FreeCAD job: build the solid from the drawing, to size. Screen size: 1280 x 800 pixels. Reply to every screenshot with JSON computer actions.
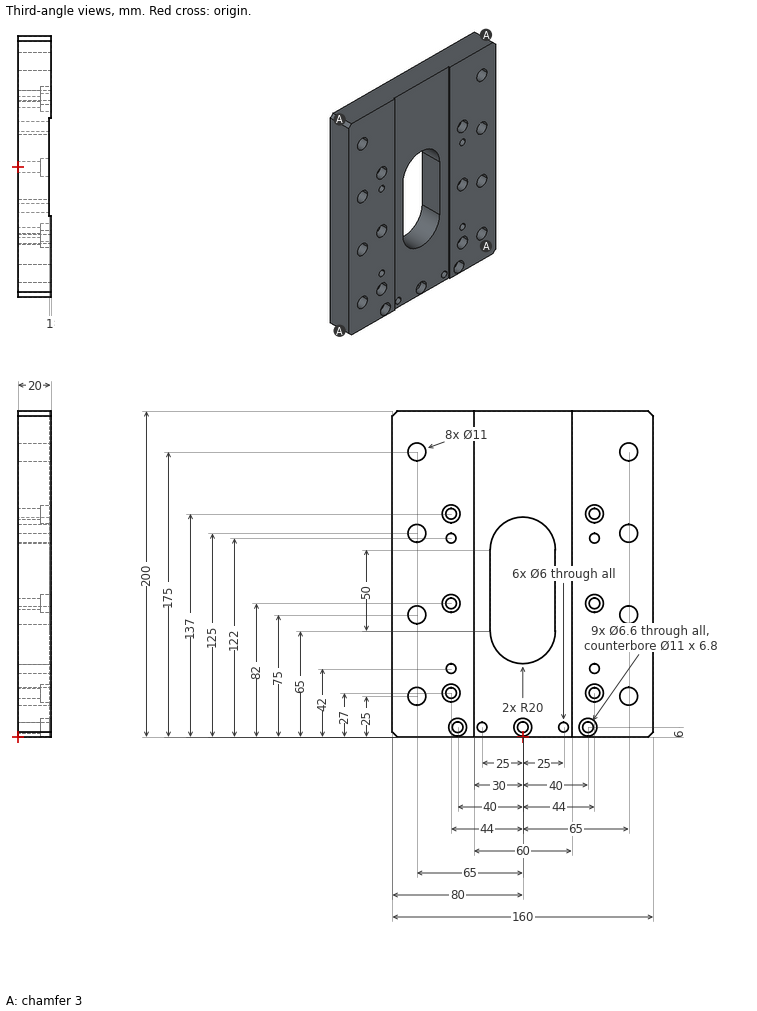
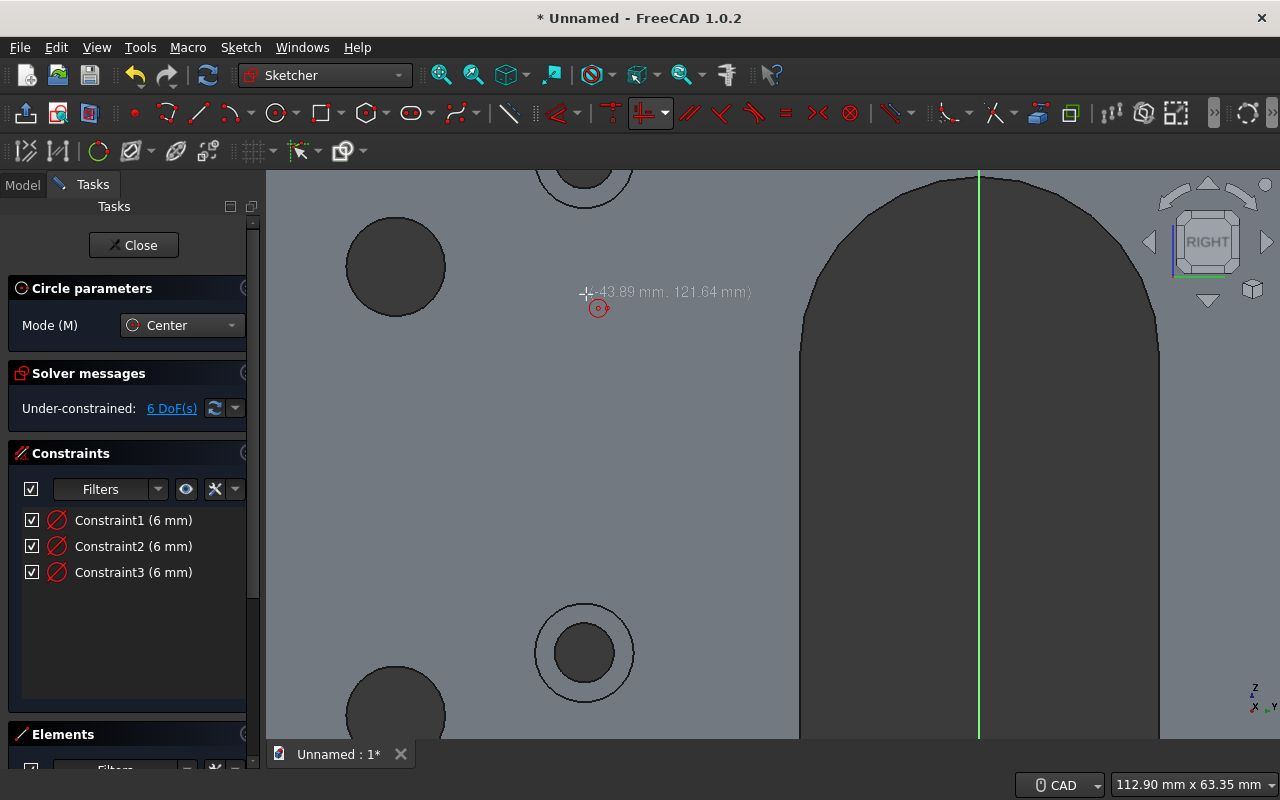
{"action": "scroll", "coordinate": [586, 294], "scroll_direction": "down", "scroll_amount": 6}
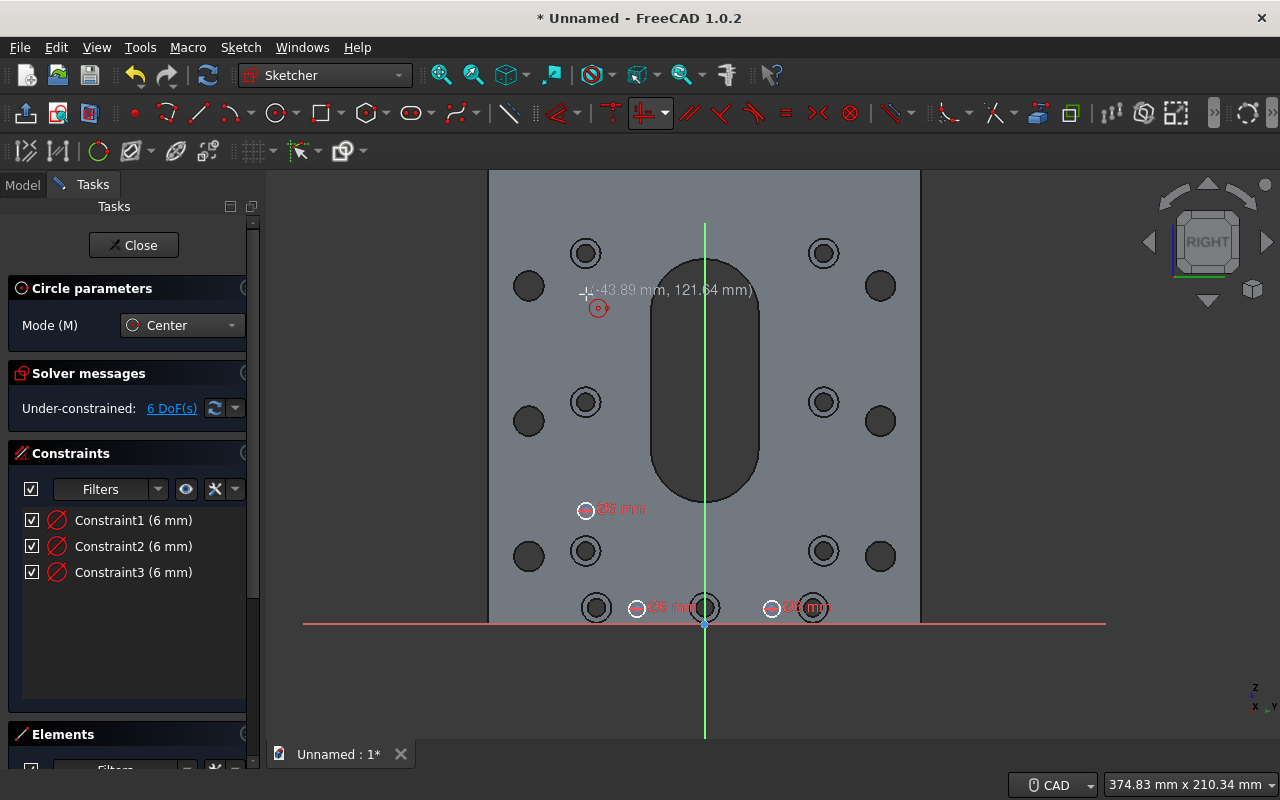
{"action": "left_click", "coordinate": [586, 294]}
{"action": "mouse_move", "coordinate": [591, 288]}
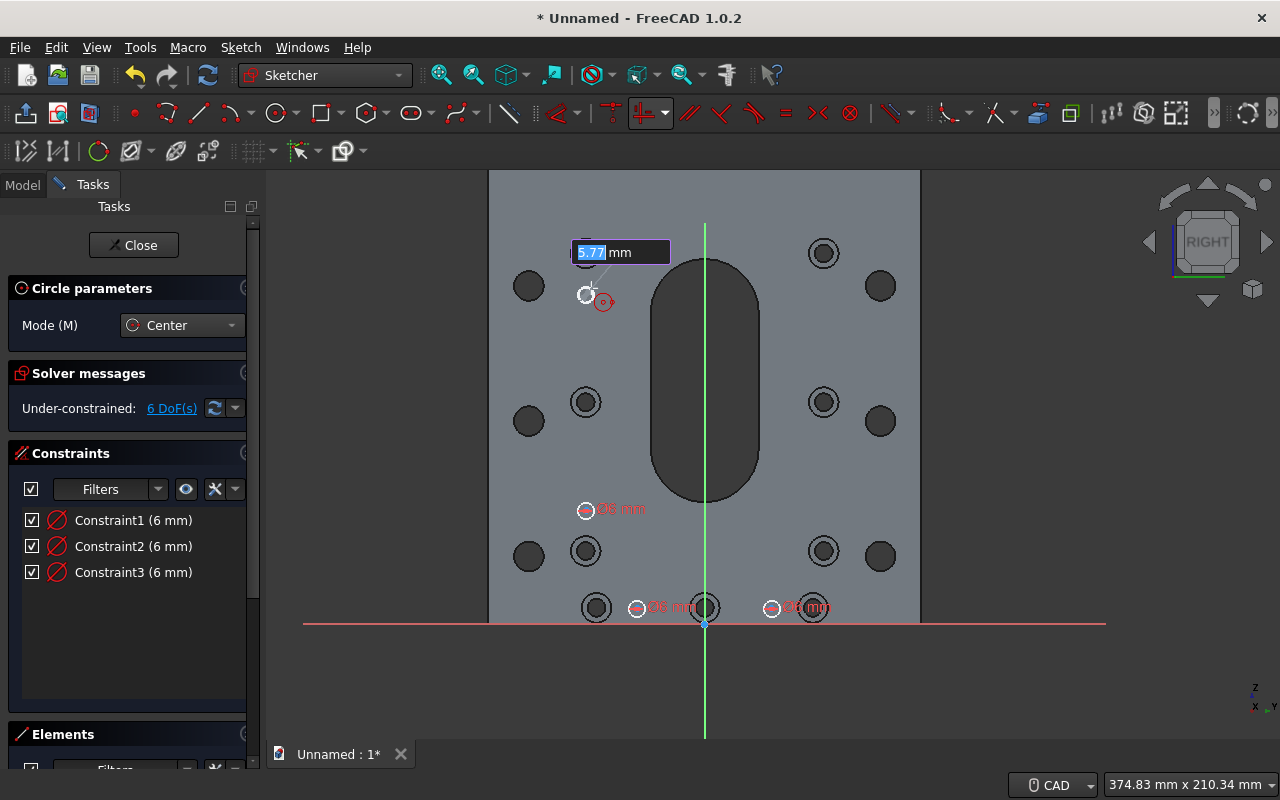
{"action": "type", "text": "6"}
{"action": "key", "text": "Return"}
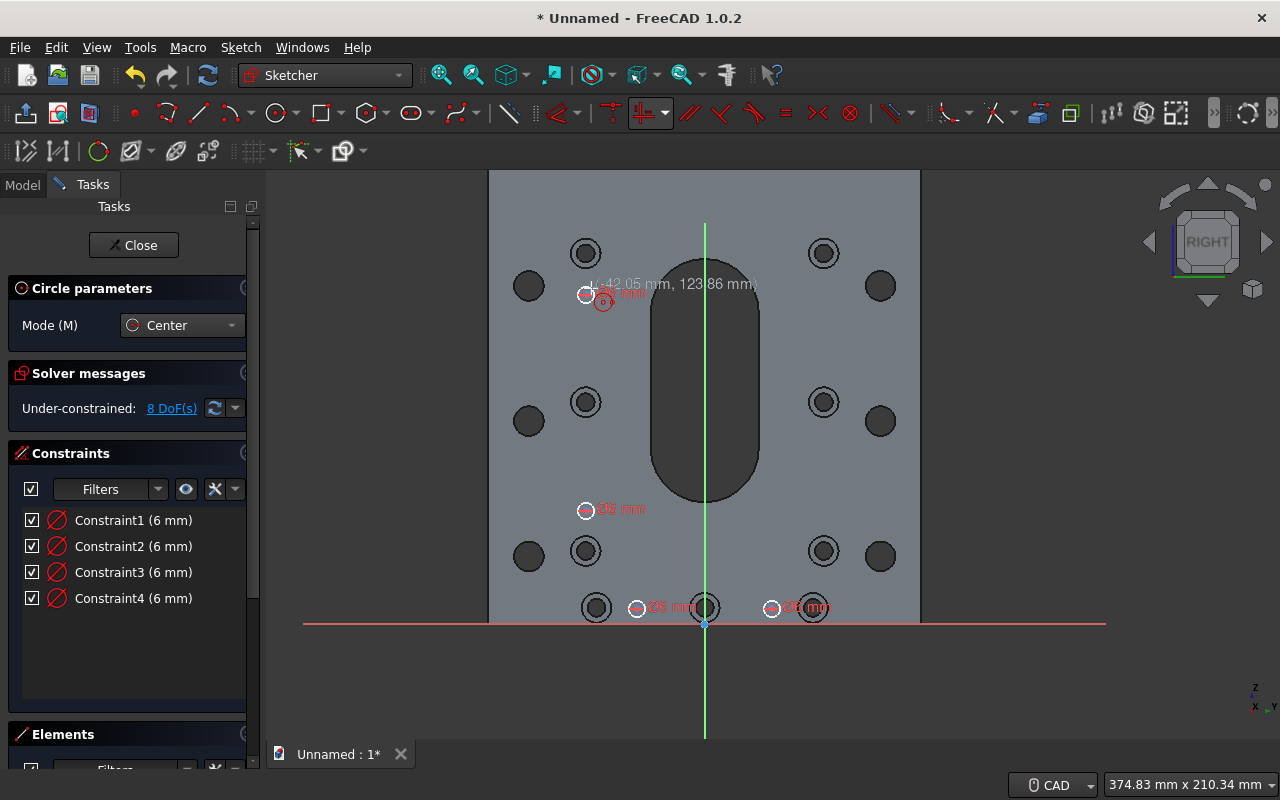
{"action": "scroll", "coordinate": [824, 294], "scroll_direction": "up", "scroll_amount": 6}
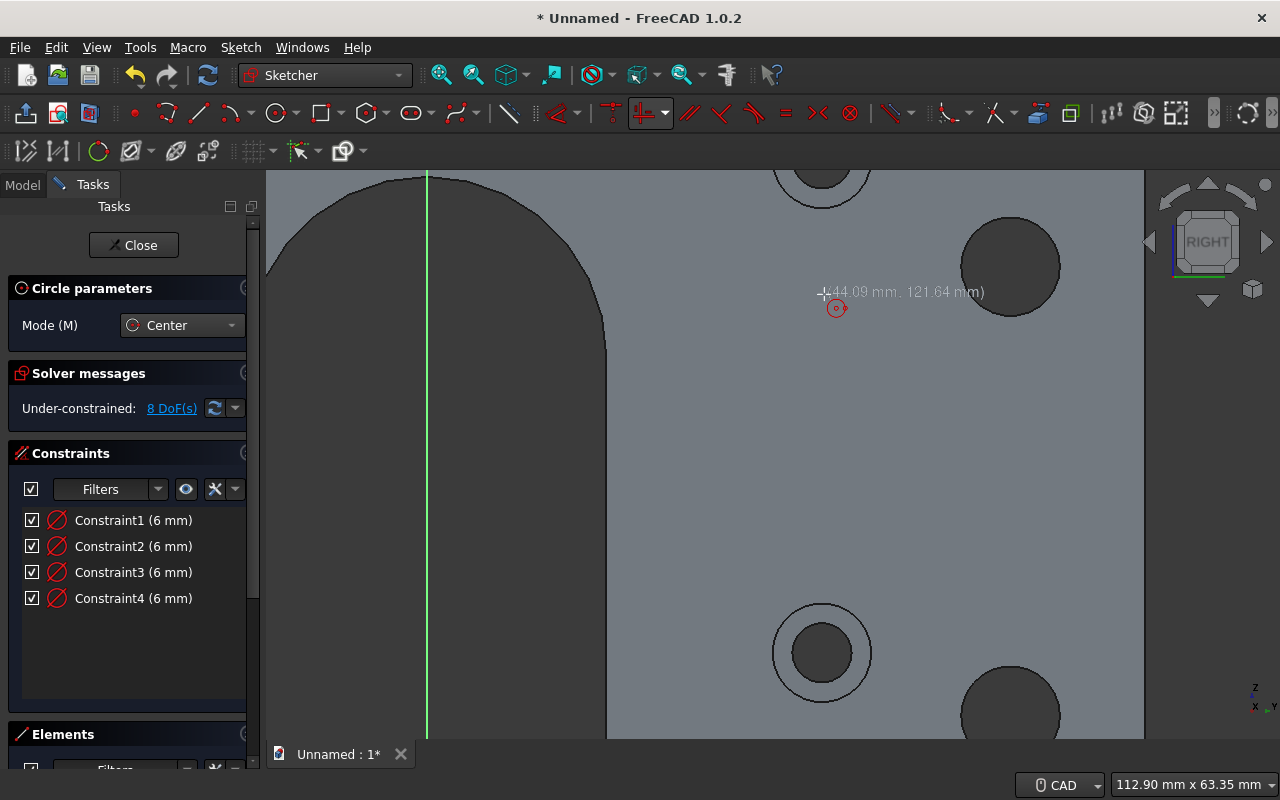
{"action": "scroll", "coordinate": [824, 294], "scroll_direction": "down", "scroll_amount": 6}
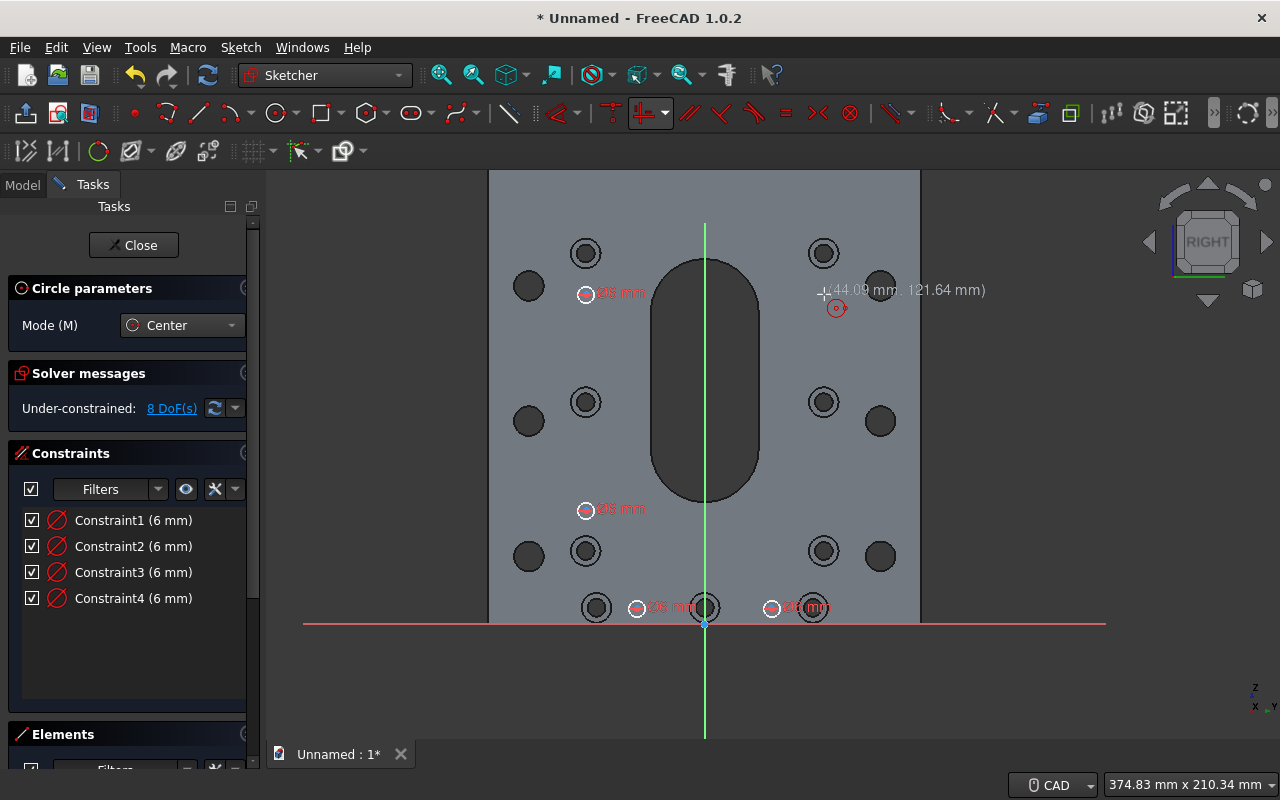
{"action": "left_click", "coordinate": [824, 294]}
{"action": "mouse_move", "coordinate": [830, 288]}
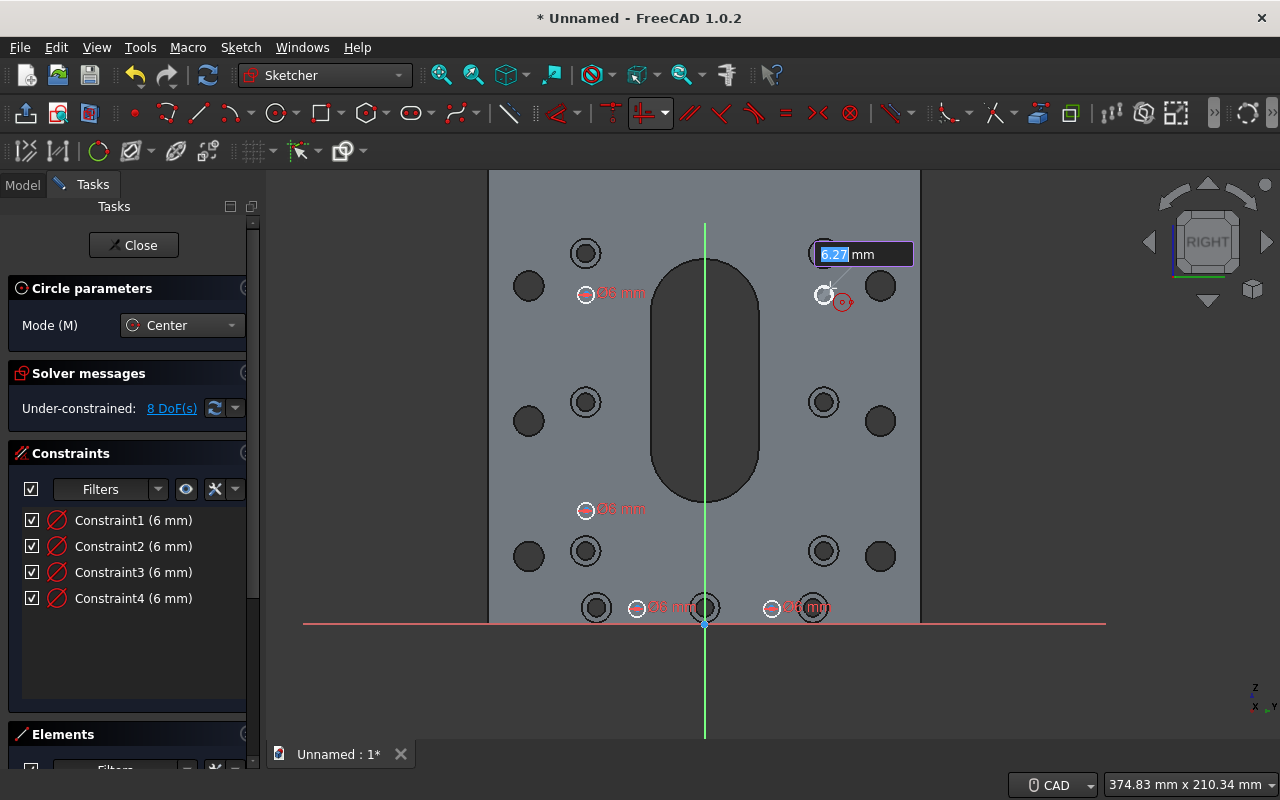
{"action": "type", "text": "6"}
{"action": "key", "text": "Return"}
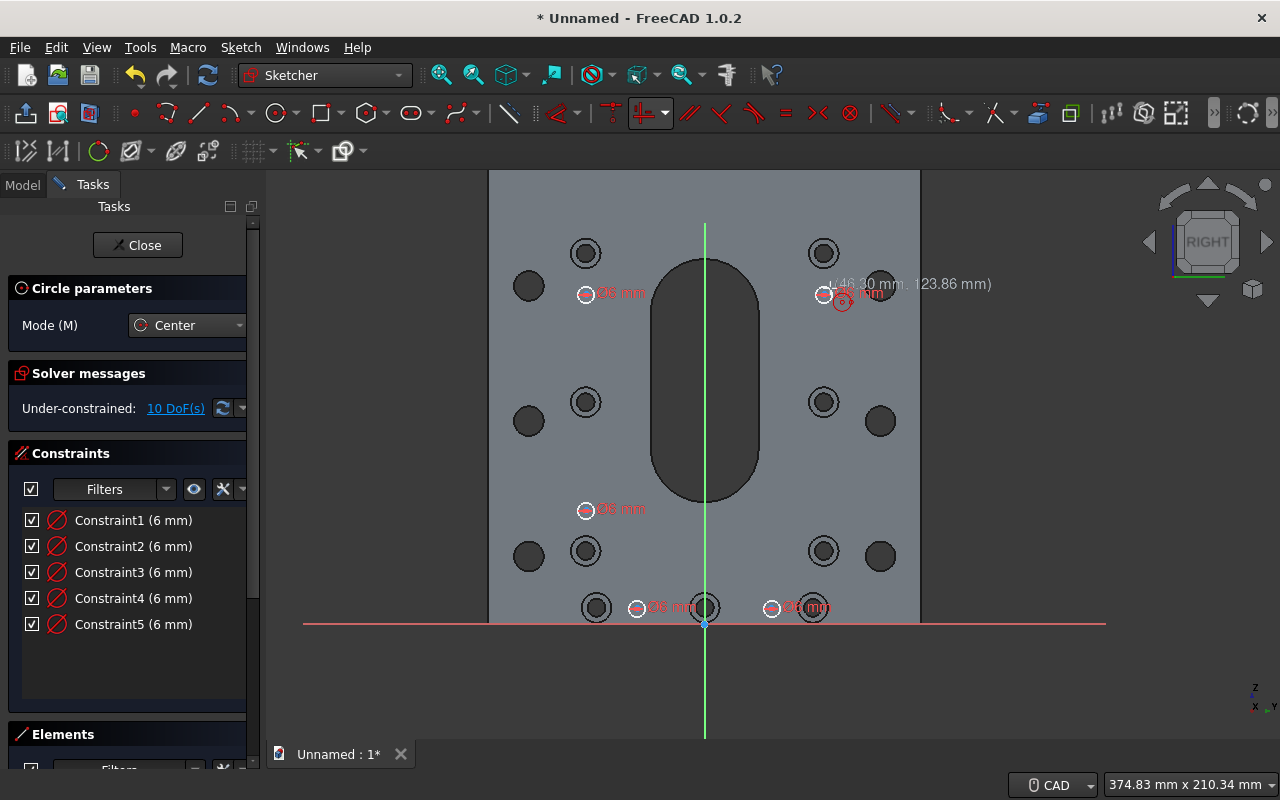
{"action": "scroll", "coordinate": [824, 510], "scroll_direction": "up", "scroll_amount": 6}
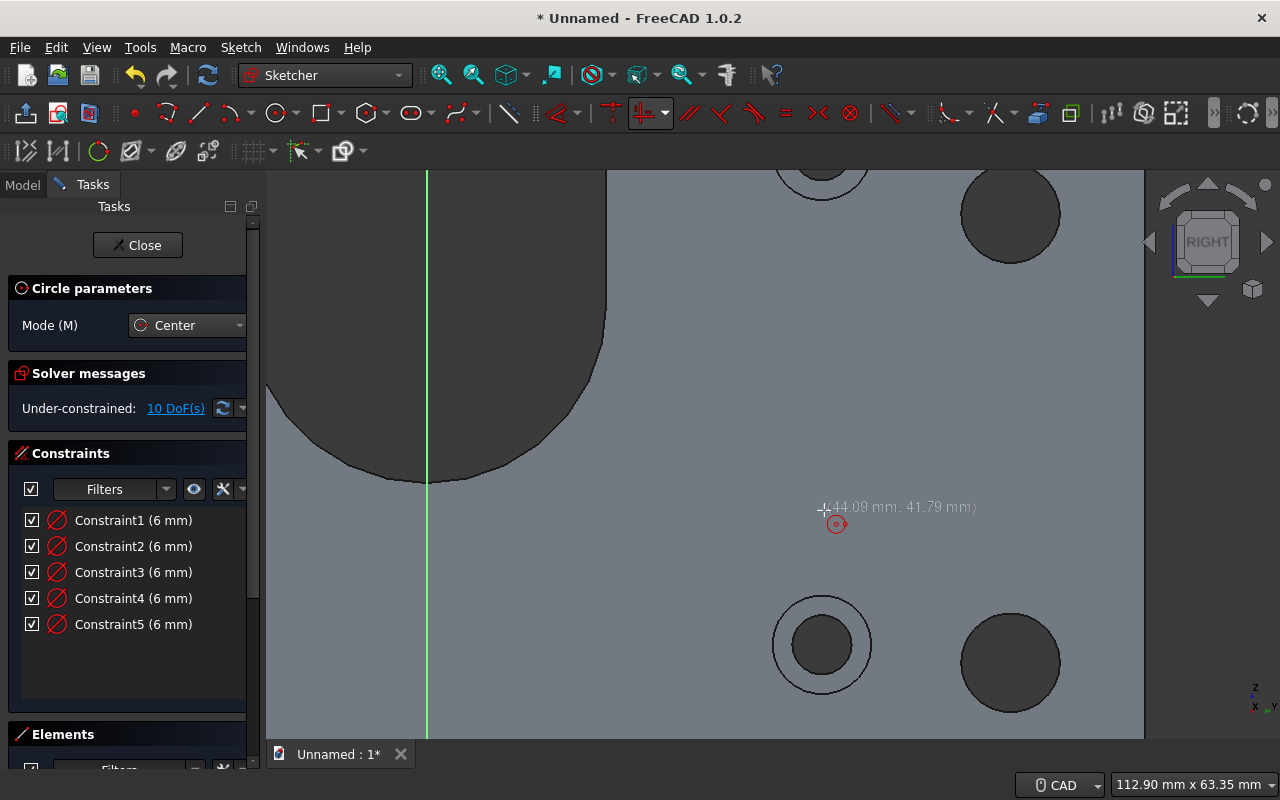
{"action": "scroll", "coordinate": [824, 510], "scroll_direction": "down", "scroll_amount": 6}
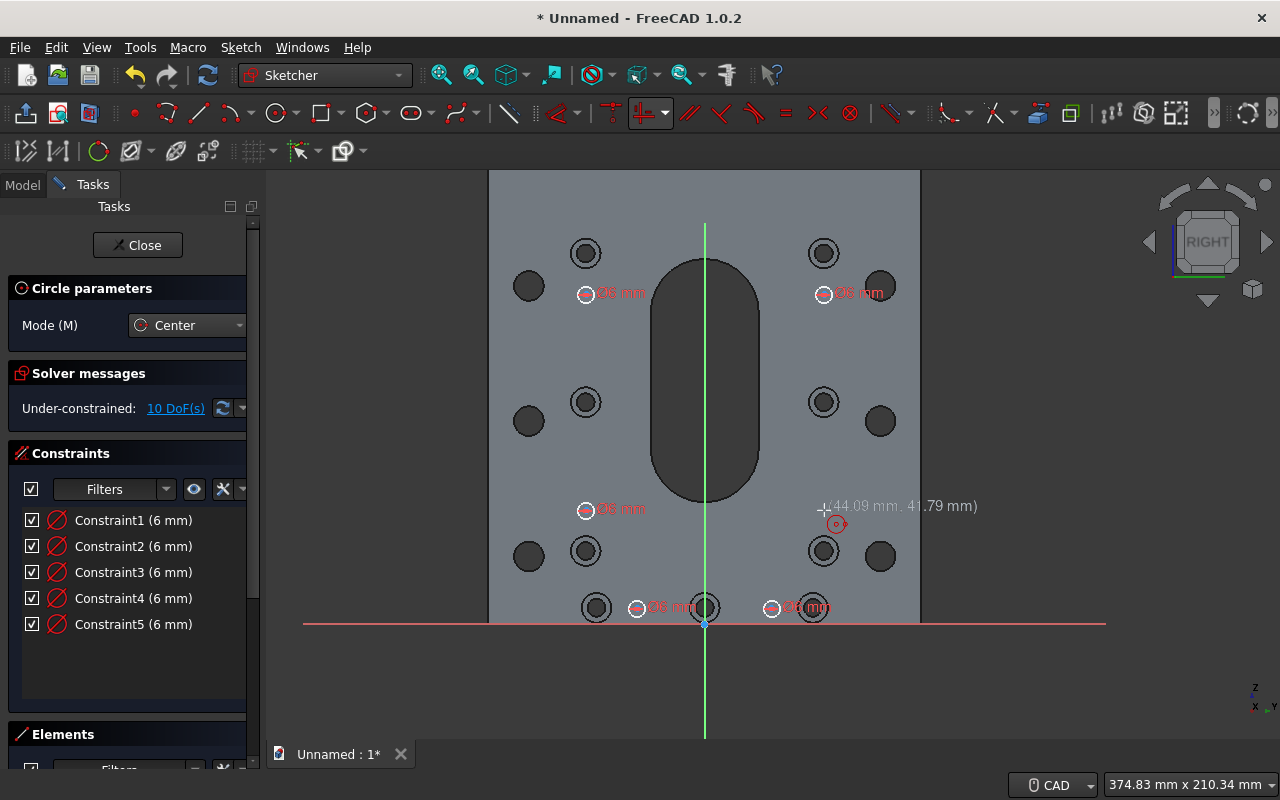
{"action": "left_click", "coordinate": [824, 510]}
{"action": "mouse_move", "coordinate": [830, 505]}